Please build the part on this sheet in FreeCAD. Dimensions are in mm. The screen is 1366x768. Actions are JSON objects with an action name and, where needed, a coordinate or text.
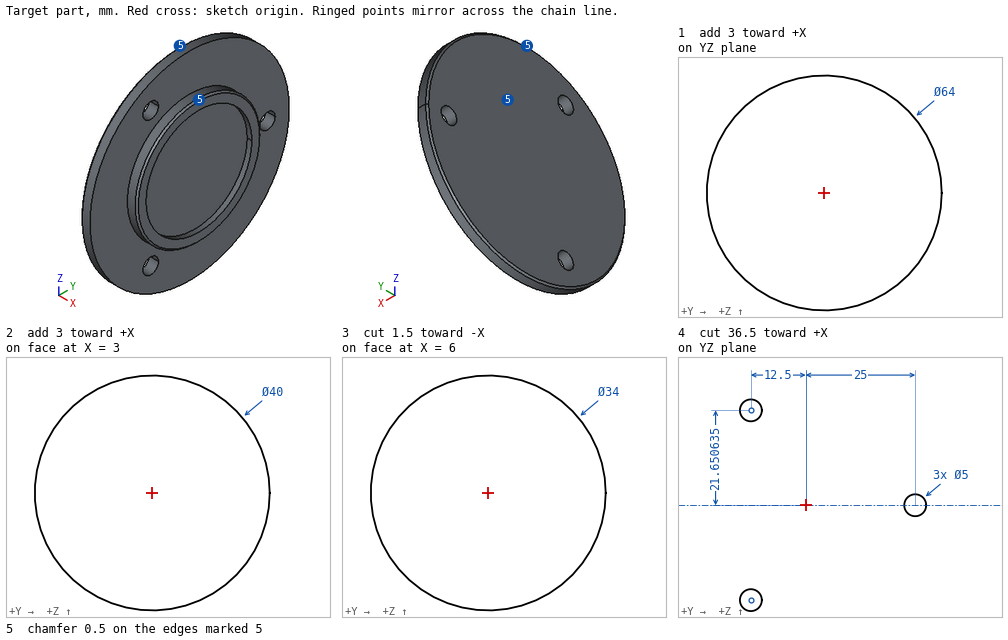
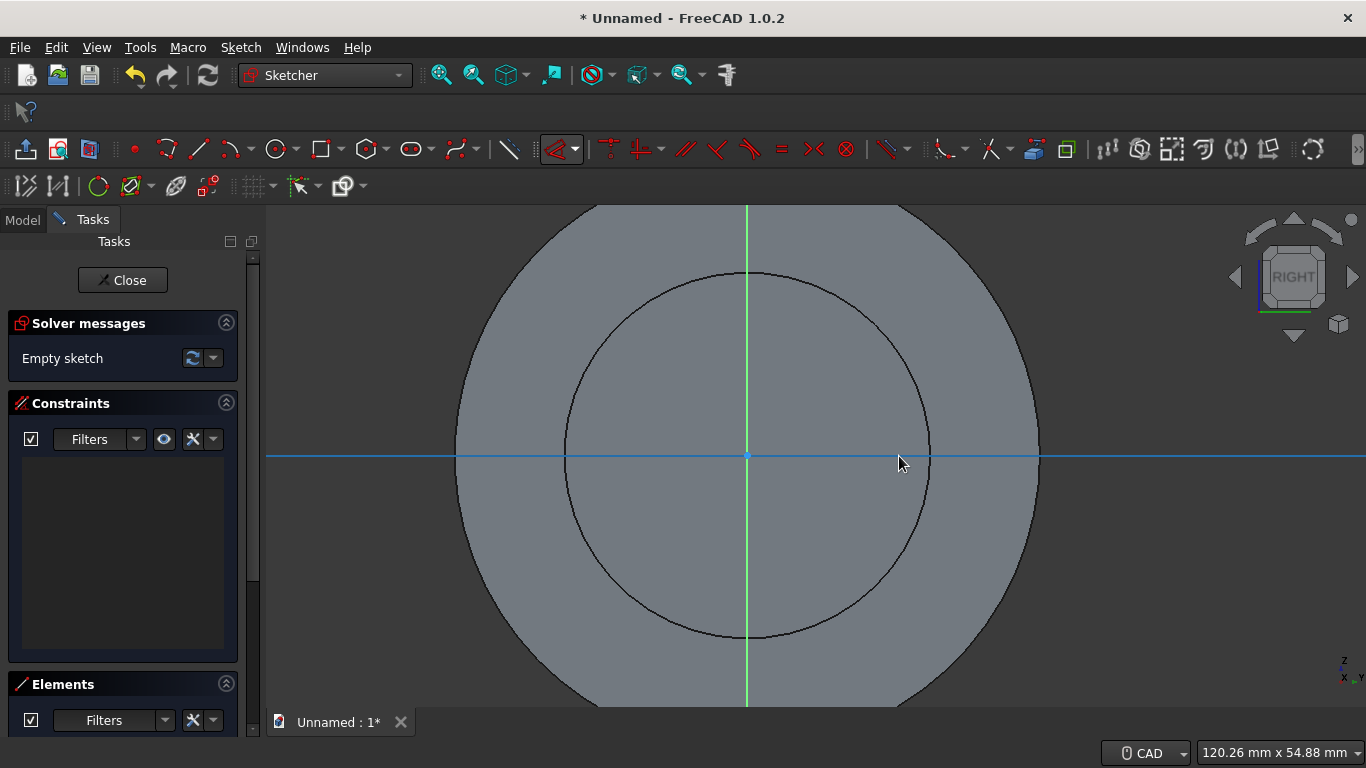
{"action": "left_click", "coordinate": [276, 150]}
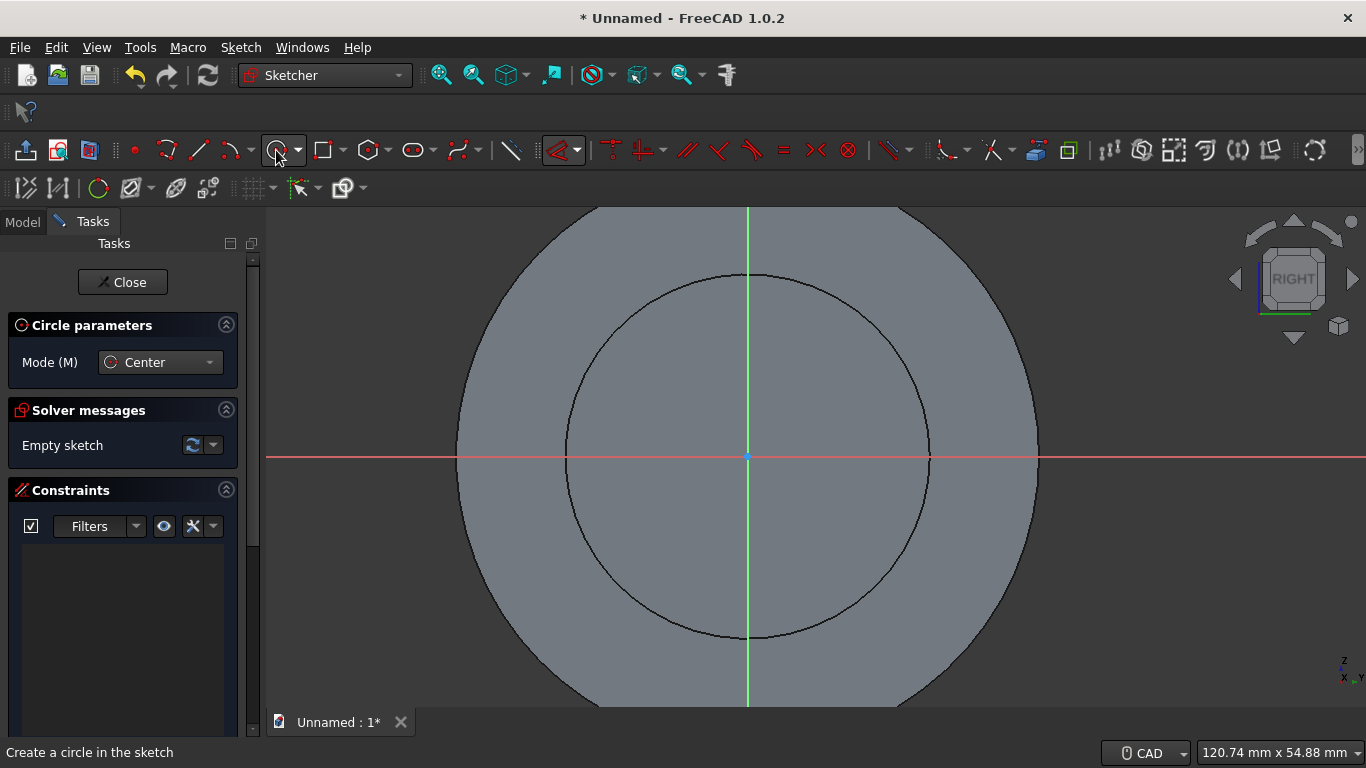
{"action": "left_click", "coordinate": [748, 457]}
{"action": "left_click", "coordinate": [857, 347]}
{"action": "key", "text": "Escape"}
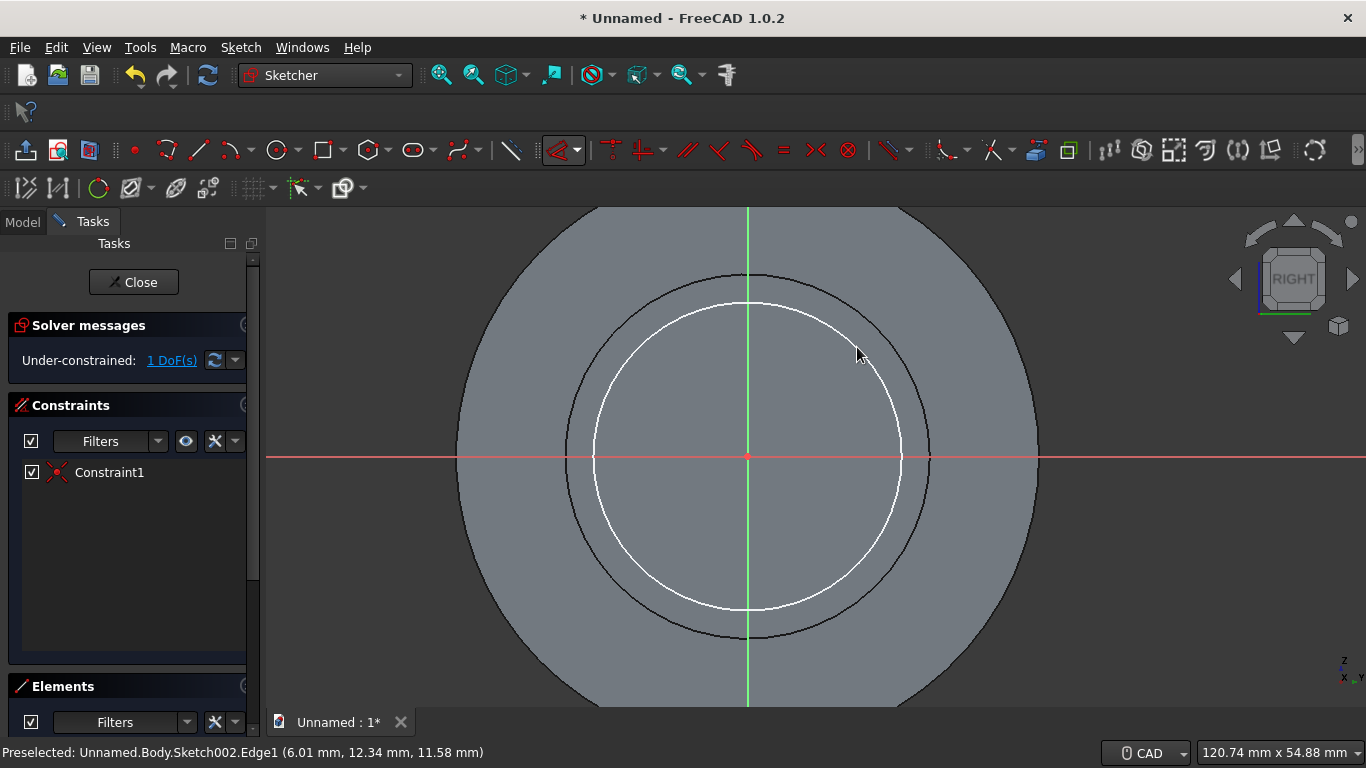
{"action": "left_click", "coordinate": [856, 347]}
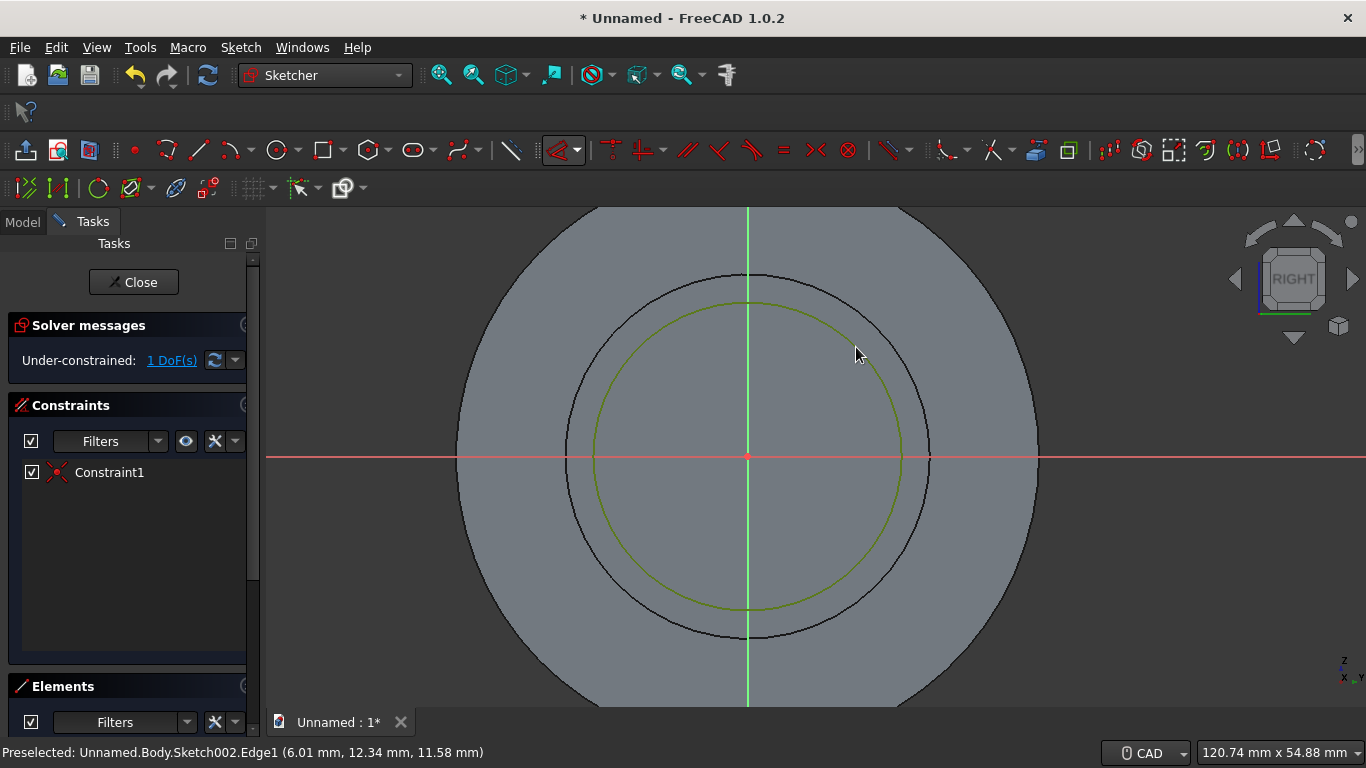
{"action": "left_click", "coordinate": [580, 150]}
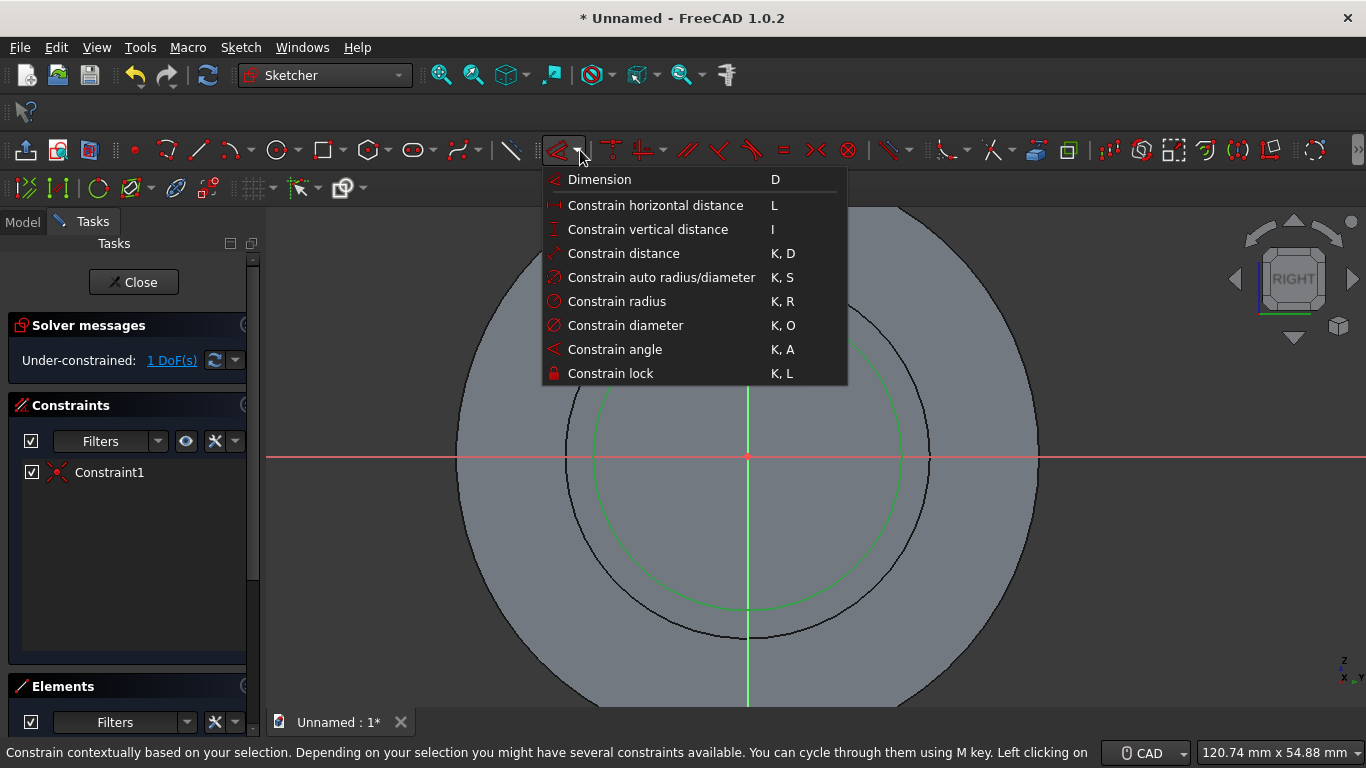
{"action": "left_click", "coordinate": [695, 325]}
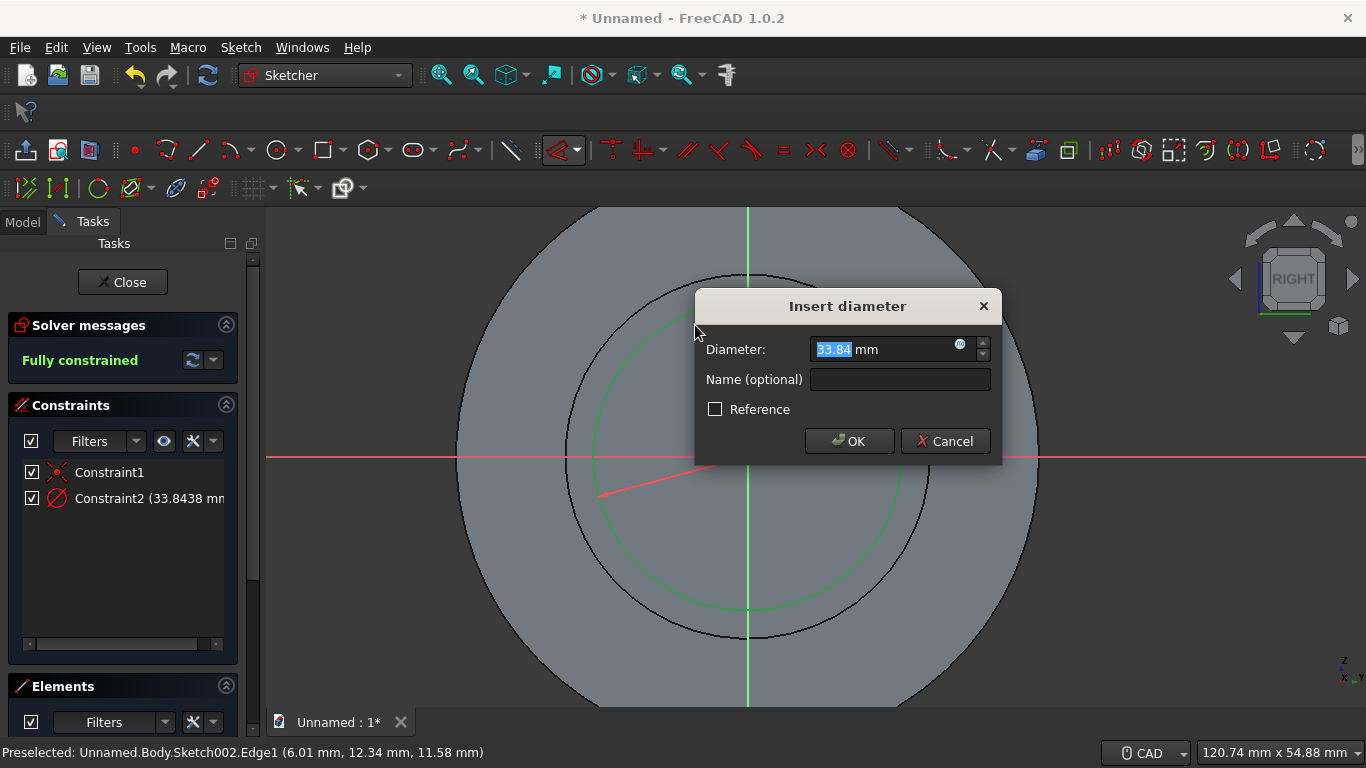
{"action": "type", "text": "34"}
{"action": "key", "text": "Return"}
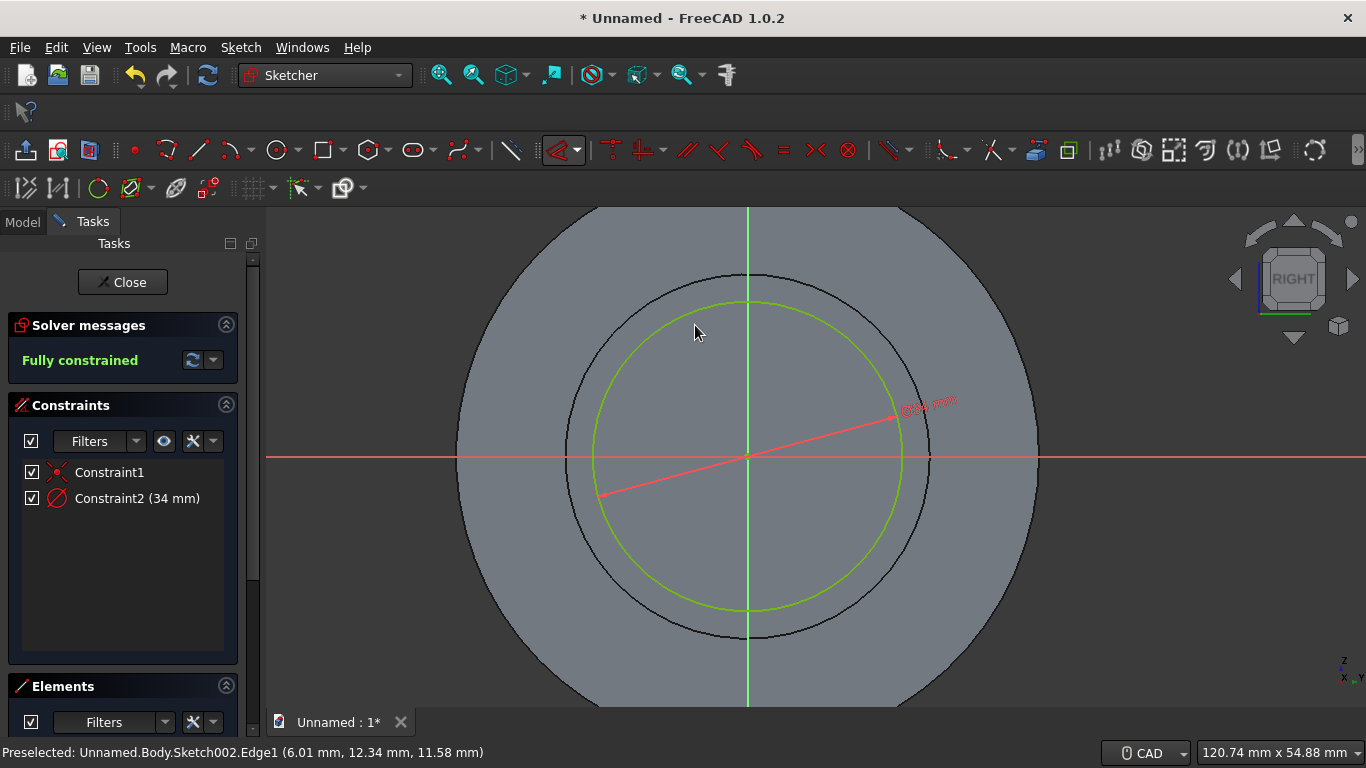
{"action": "left_click", "coordinate": [123, 282]}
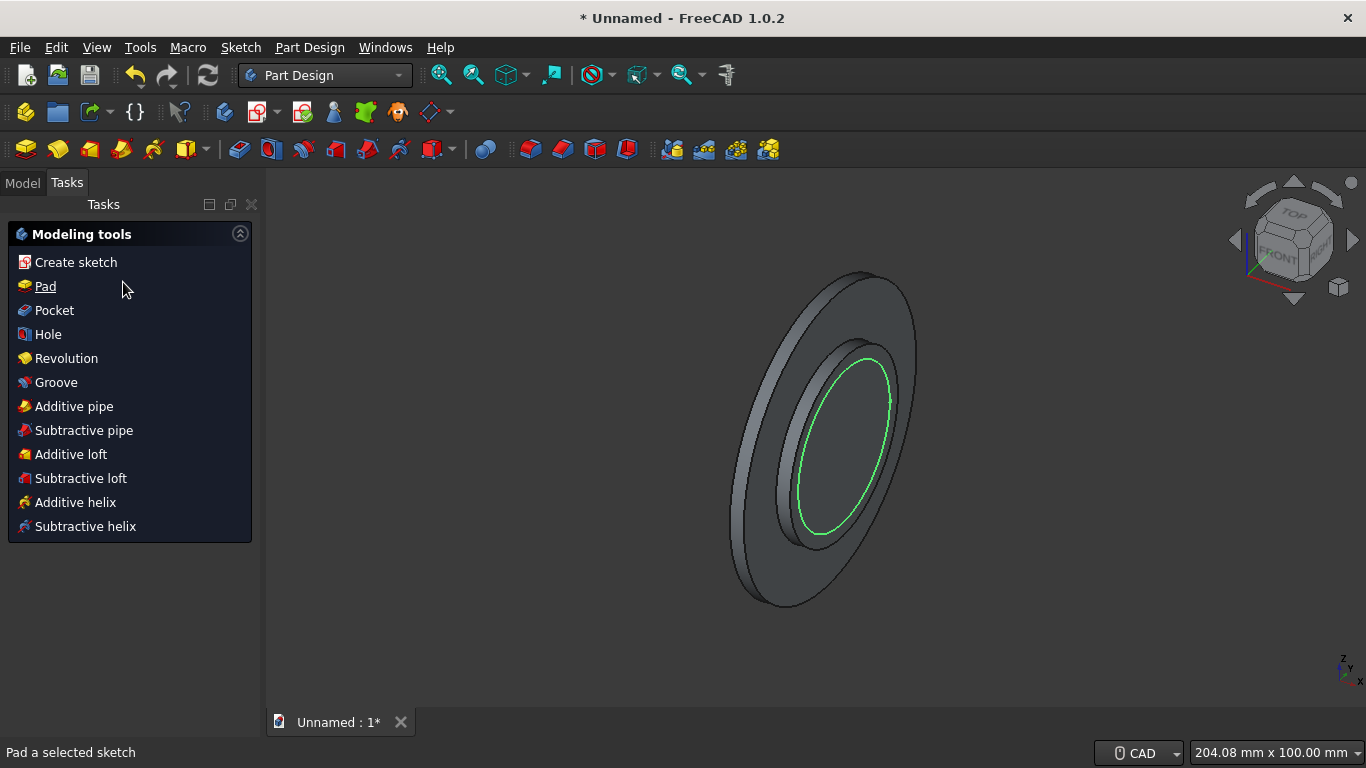
{"action": "left_click", "coordinate": [240, 150]}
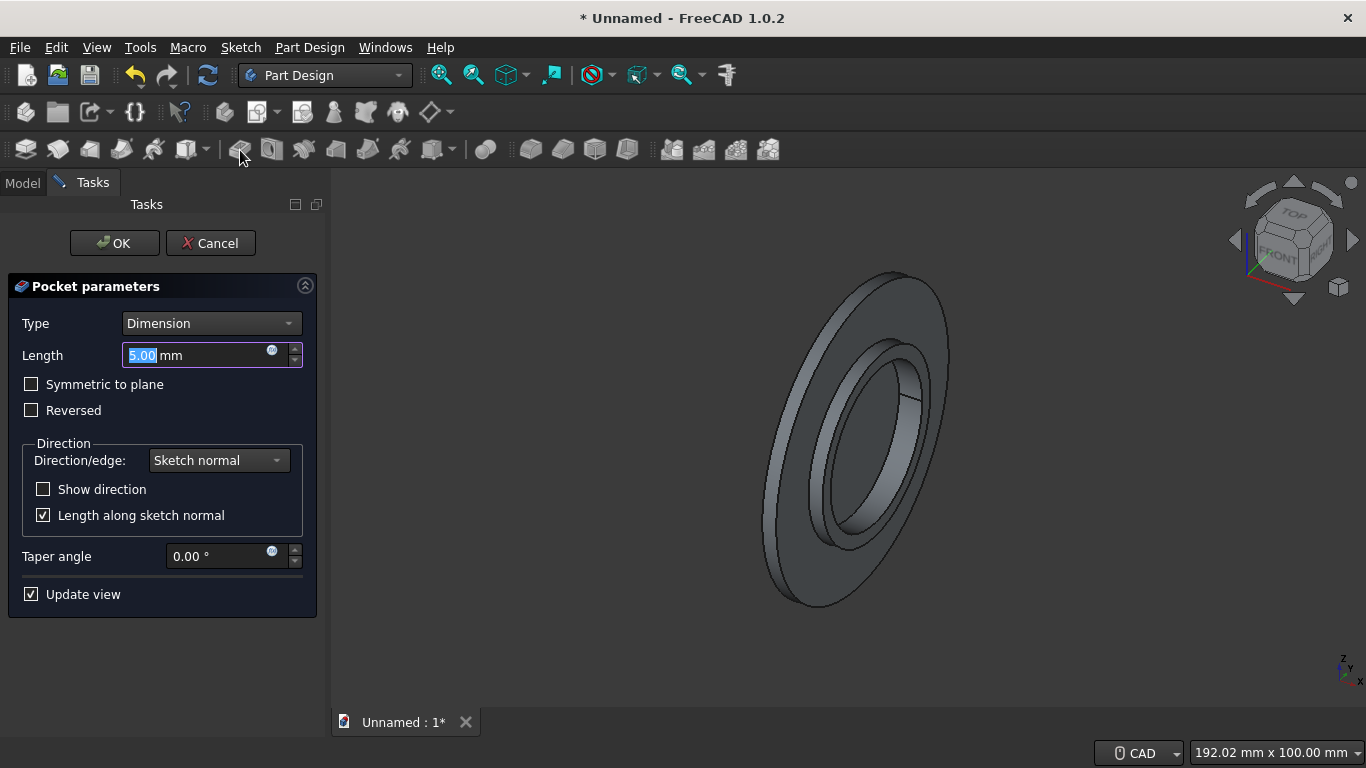
{"action": "type", "text": "1.5"}
{"action": "key", "text": "Tab"}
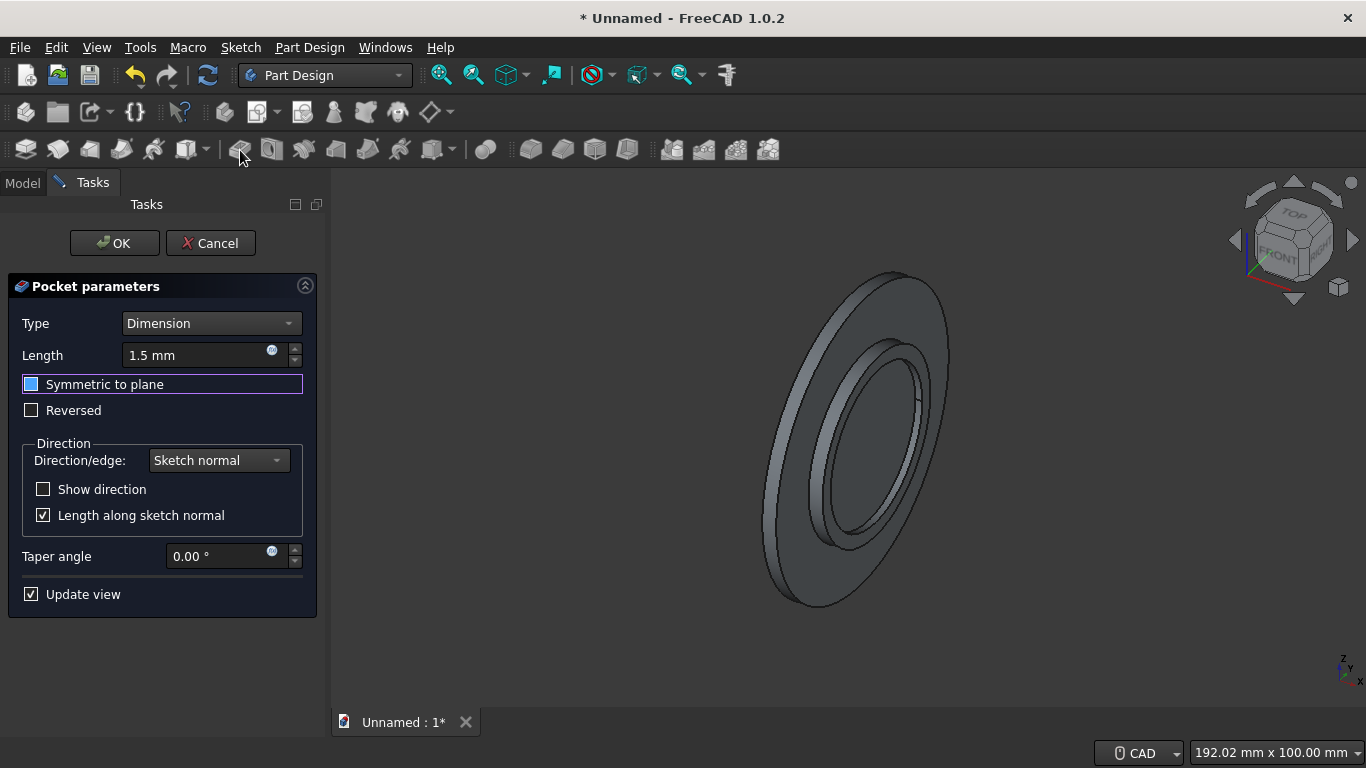
{"action": "left_click", "coordinate": [115, 243]}